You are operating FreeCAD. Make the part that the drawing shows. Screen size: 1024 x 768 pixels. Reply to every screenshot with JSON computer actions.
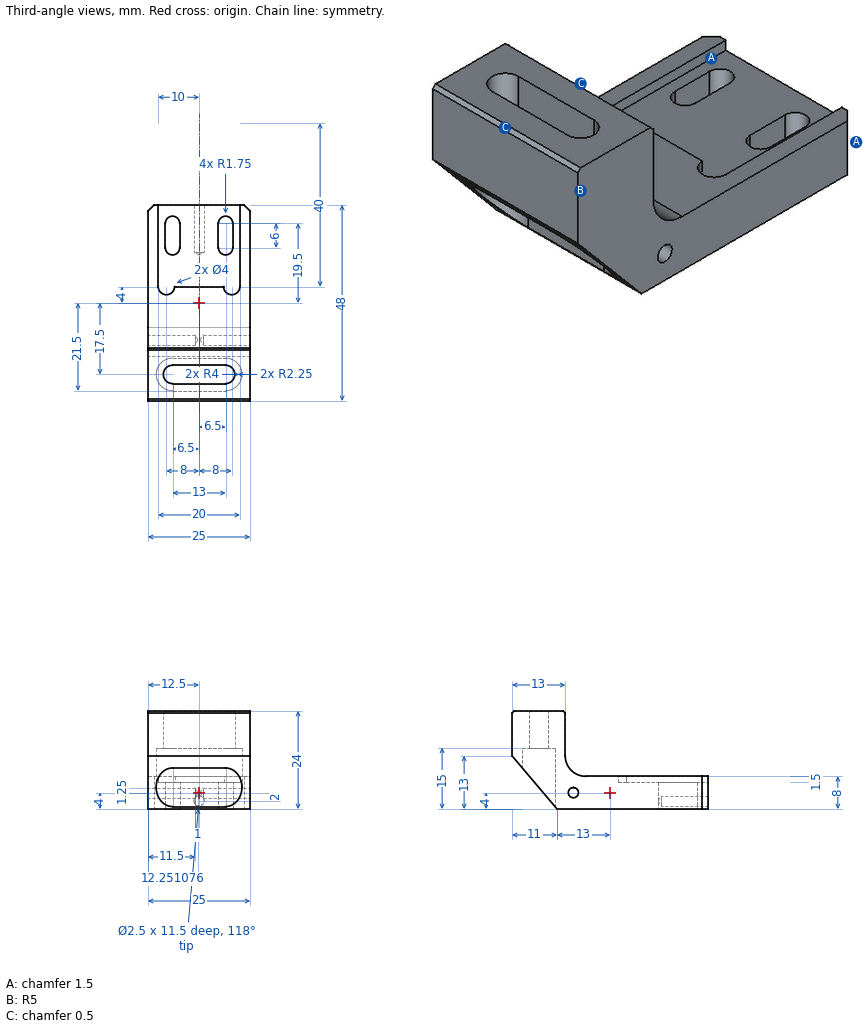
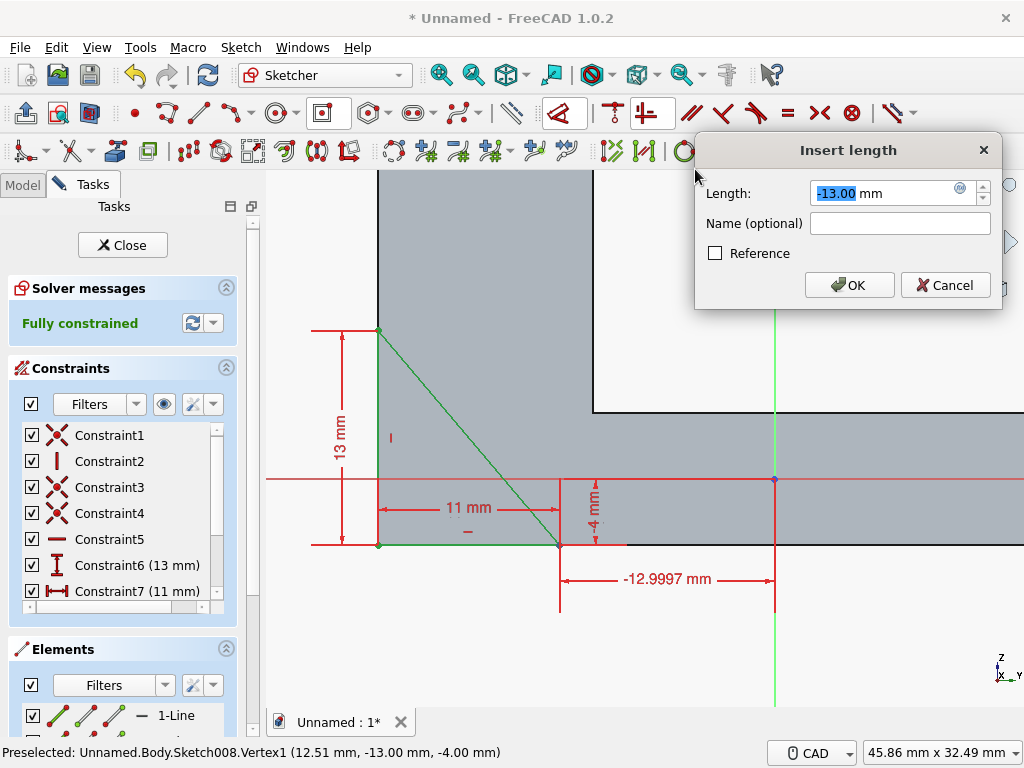
{"action": "type", "text": "-13"}
{"action": "key", "text": "Return"}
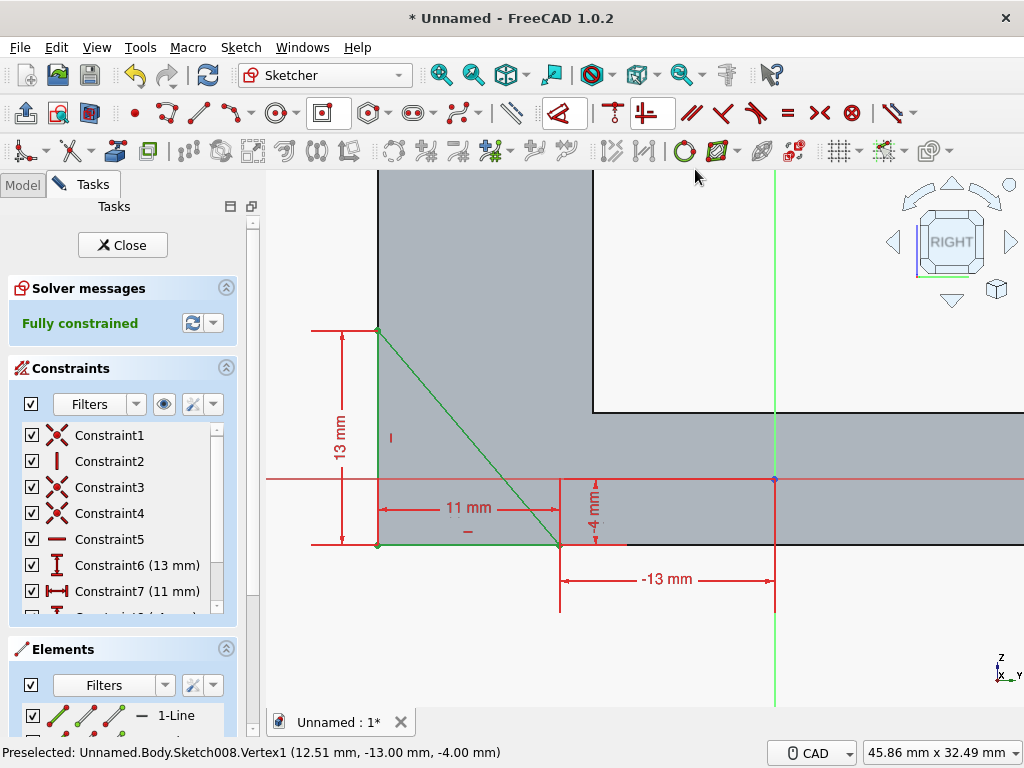
{"action": "left_click", "coordinate": [123, 245]}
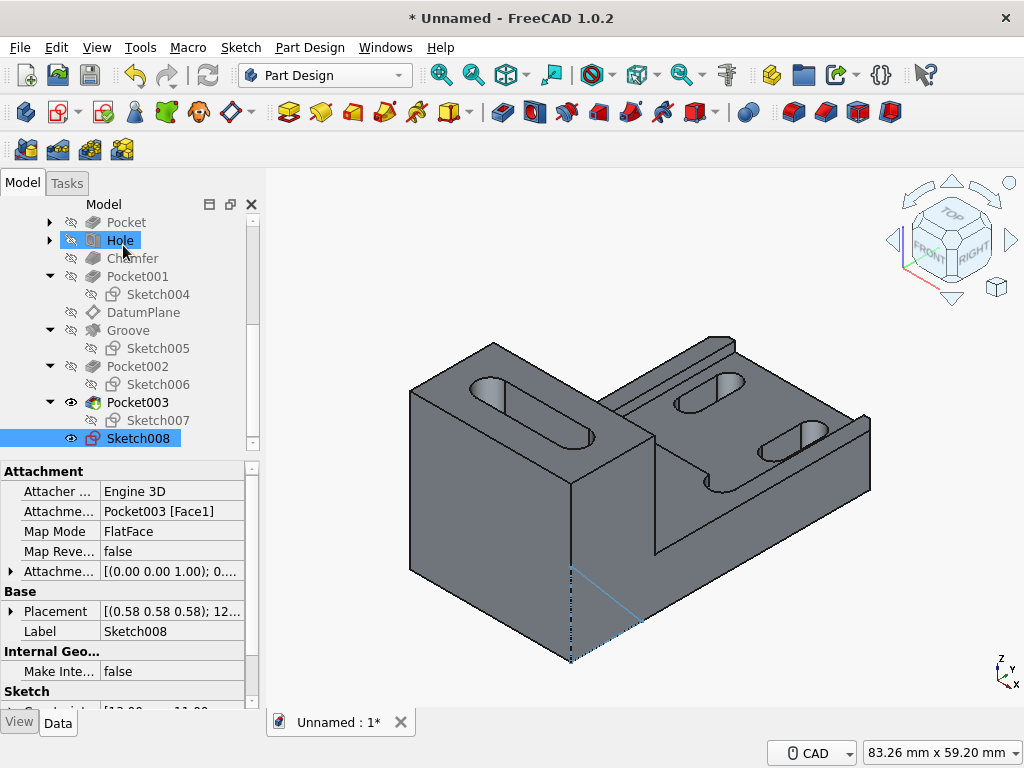
{"action": "left_click", "coordinate": [504, 112]}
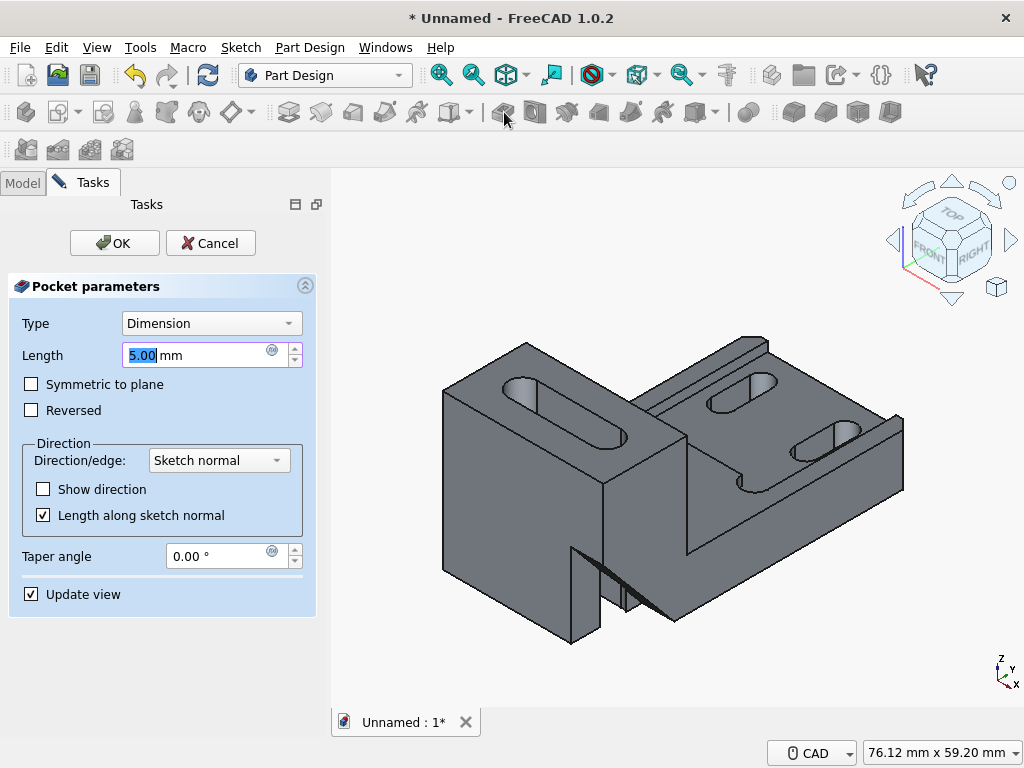
{"action": "left_click", "coordinate": [212, 324]}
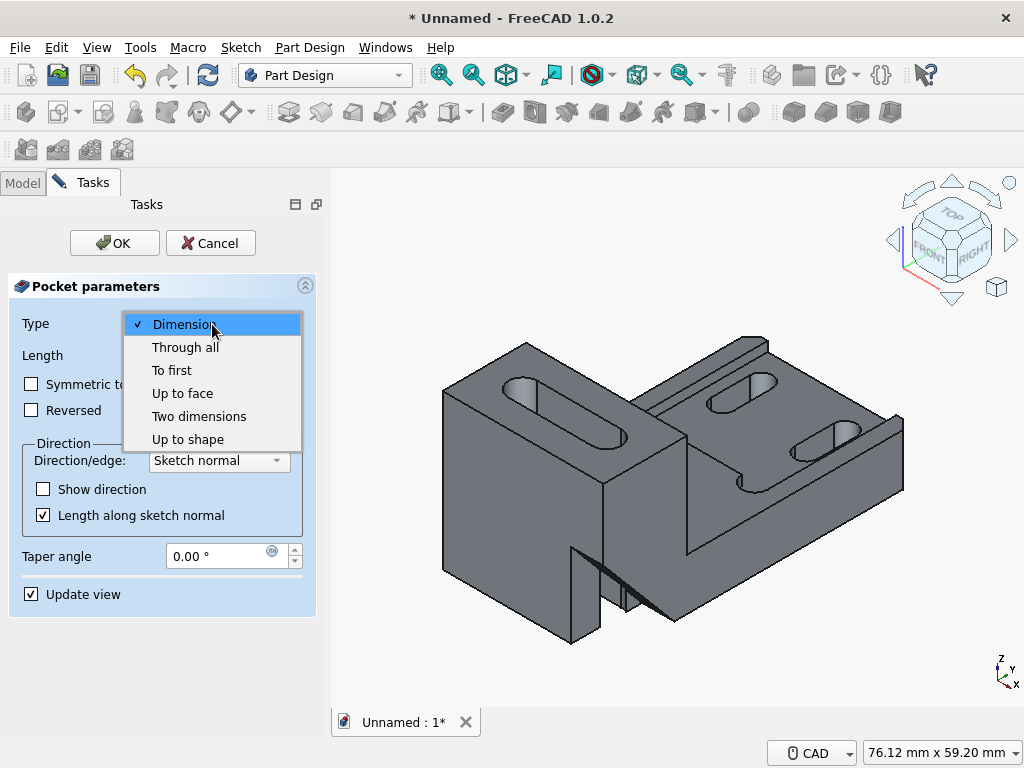
{"action": "left_click", "coordinate": [212, 348]}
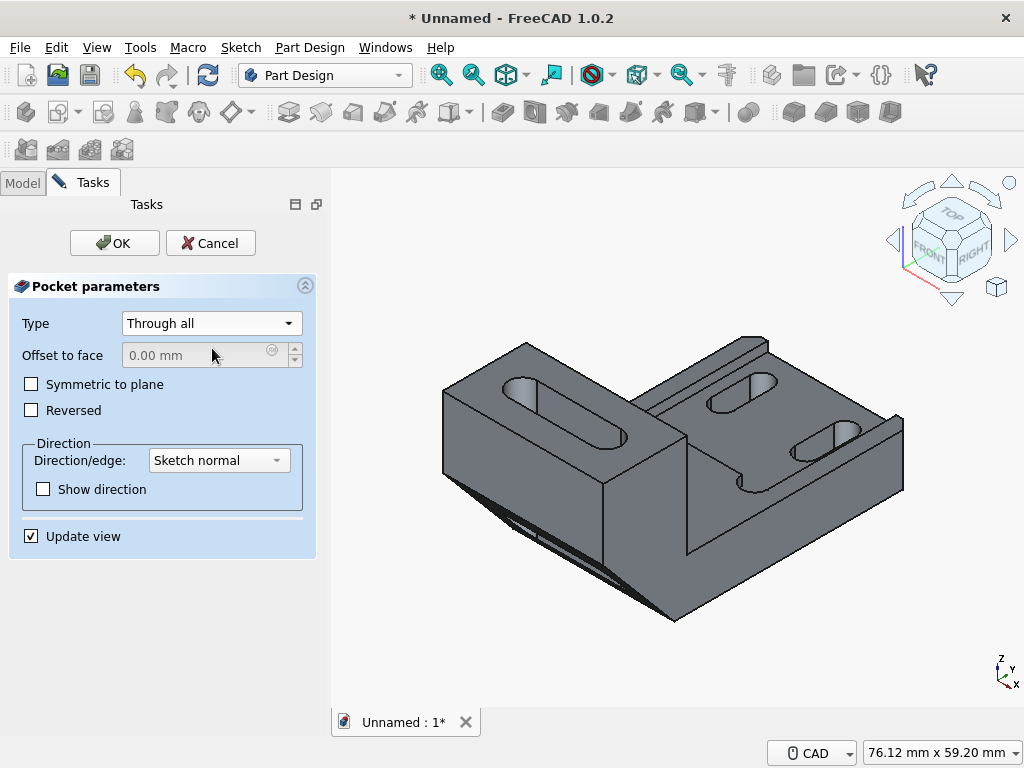
{"action": "left_click", "coordinate": [115, 243]}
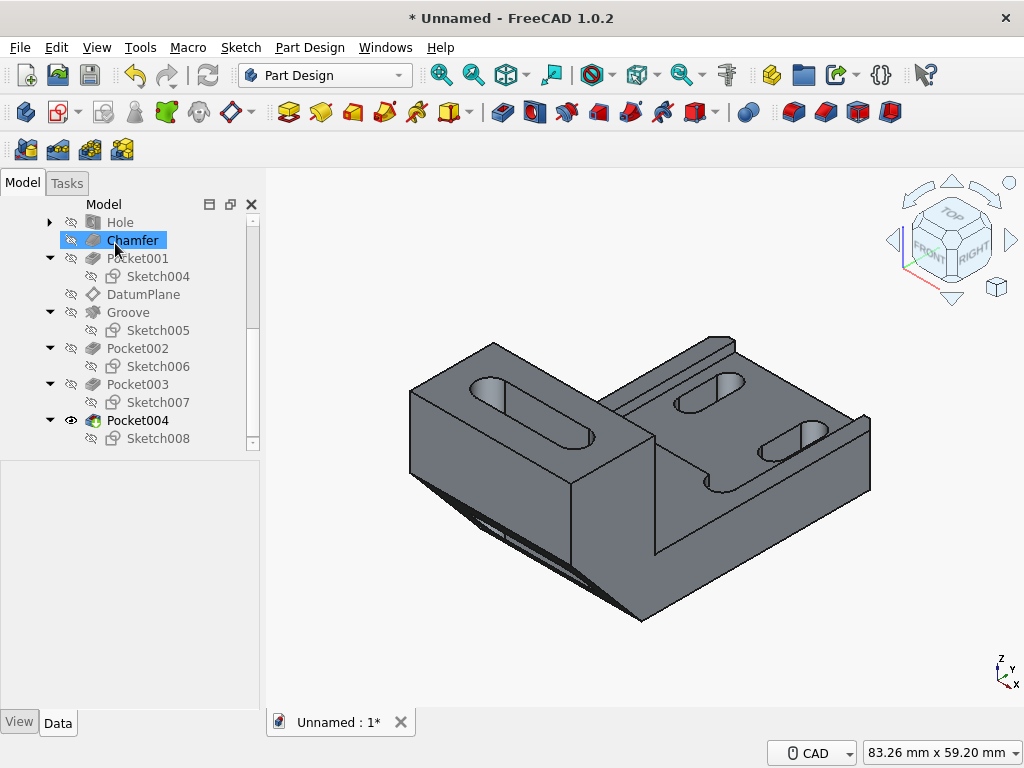
{"action": "key", "text": "5"}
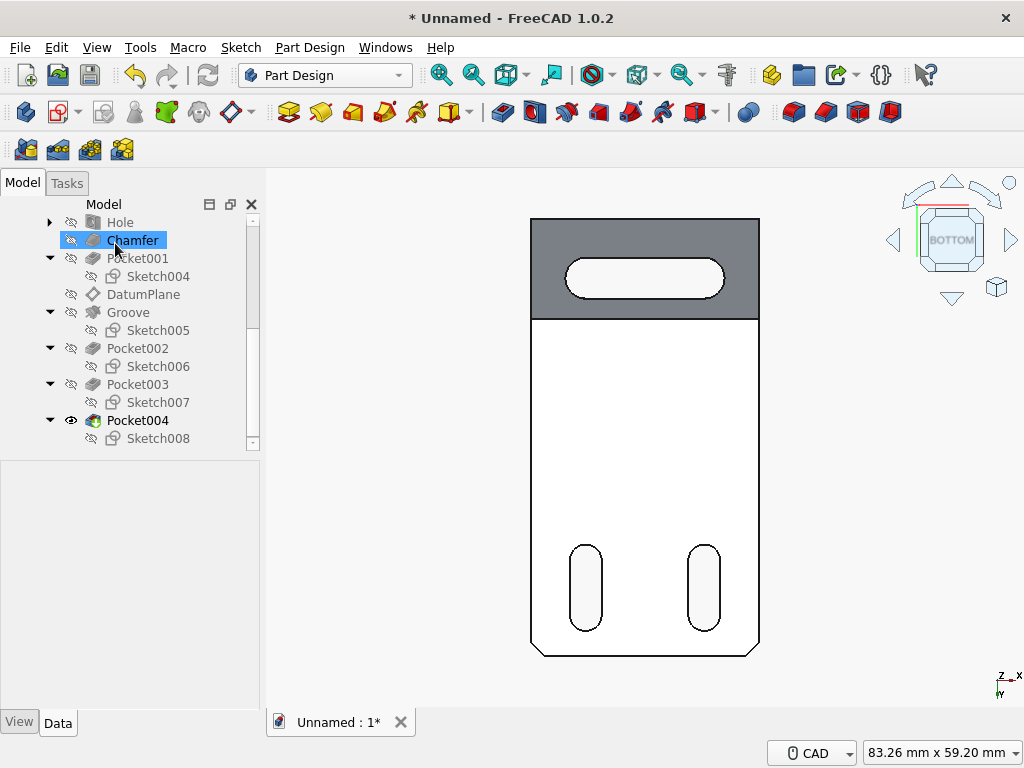
{"action": "left_click", "coordinate": [645, 438]}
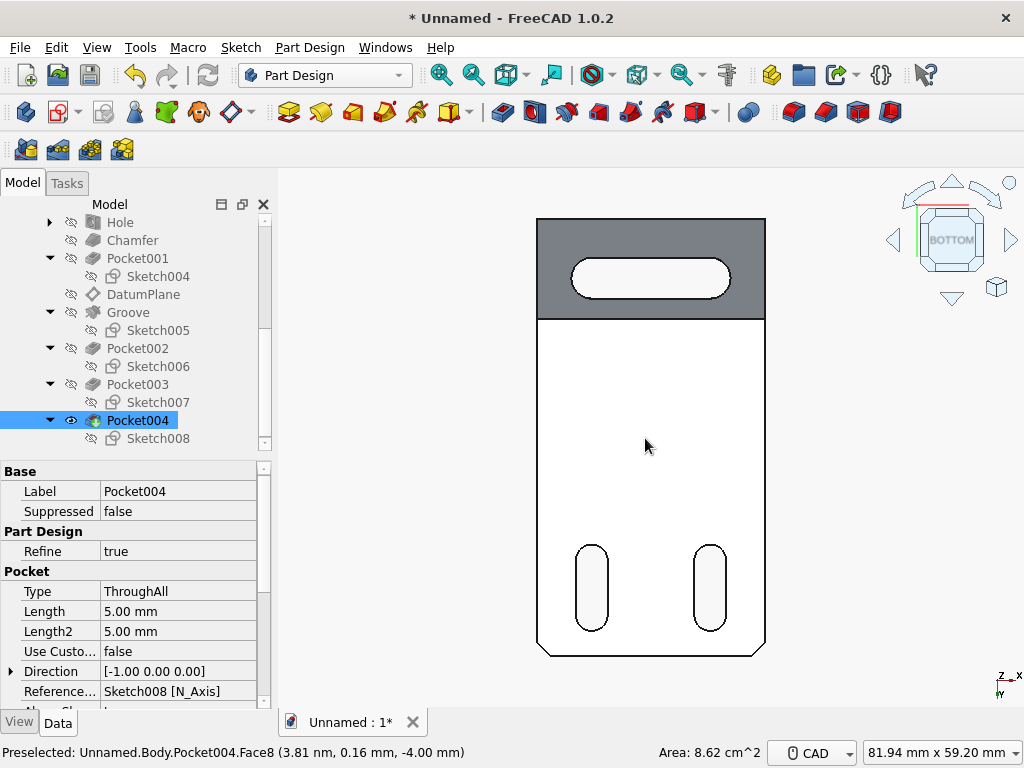
{"action": "left_click", "coordinate": [58, 112]}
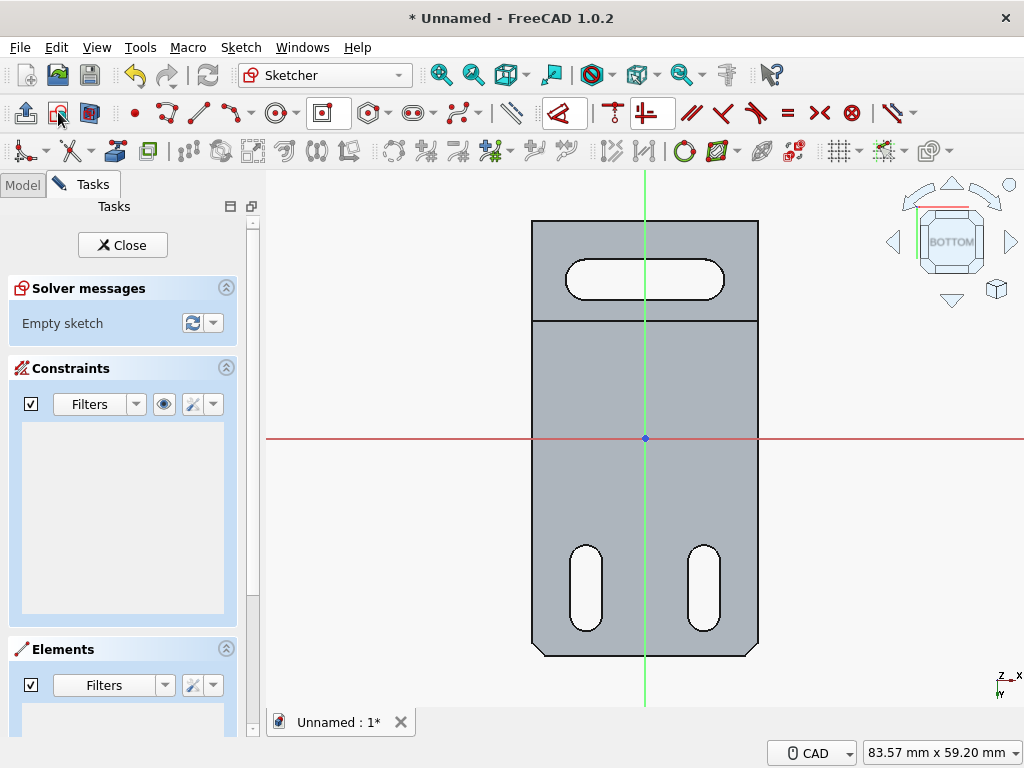
{"action": "scroll", "coordinate": [728, 222], "scroll_direction": "up", "scroll_amount": 3}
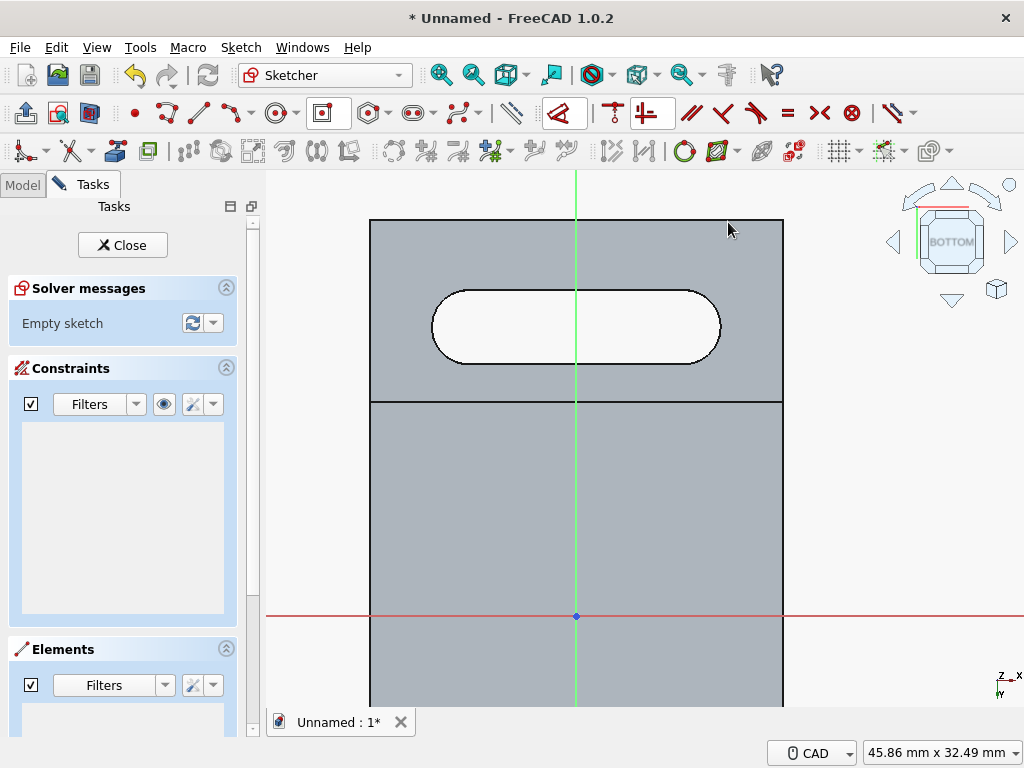
{"action": "left_click", "coordinate": [414, 114]}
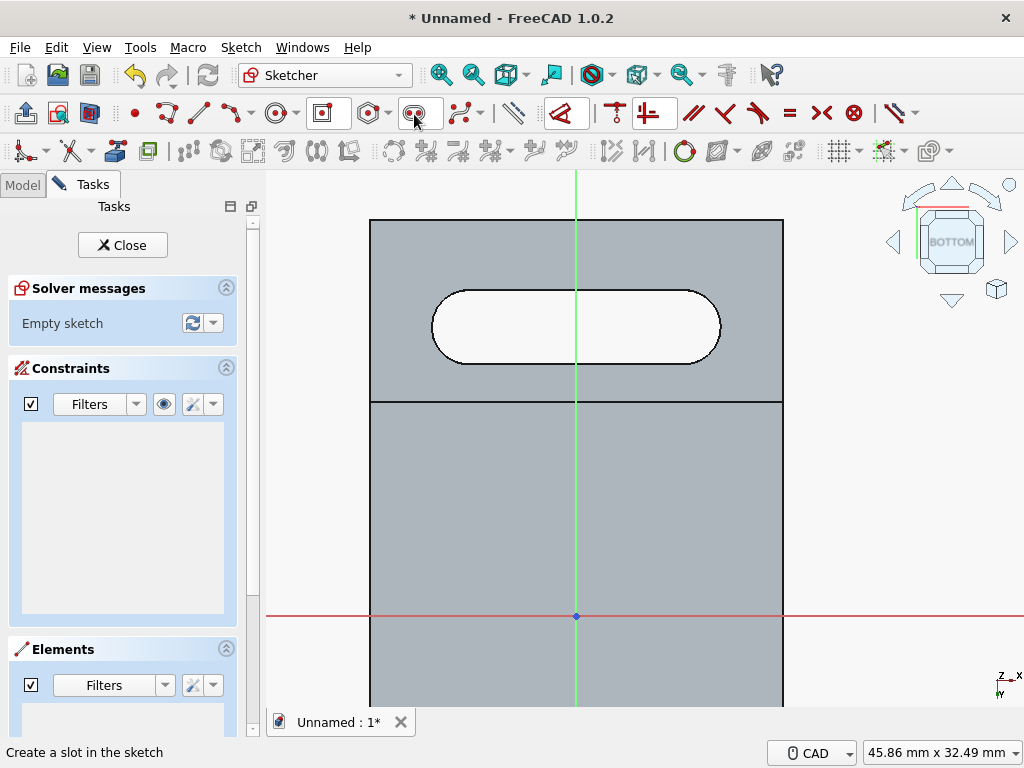
{"action": "left_click", "coordinate": [469, 327]}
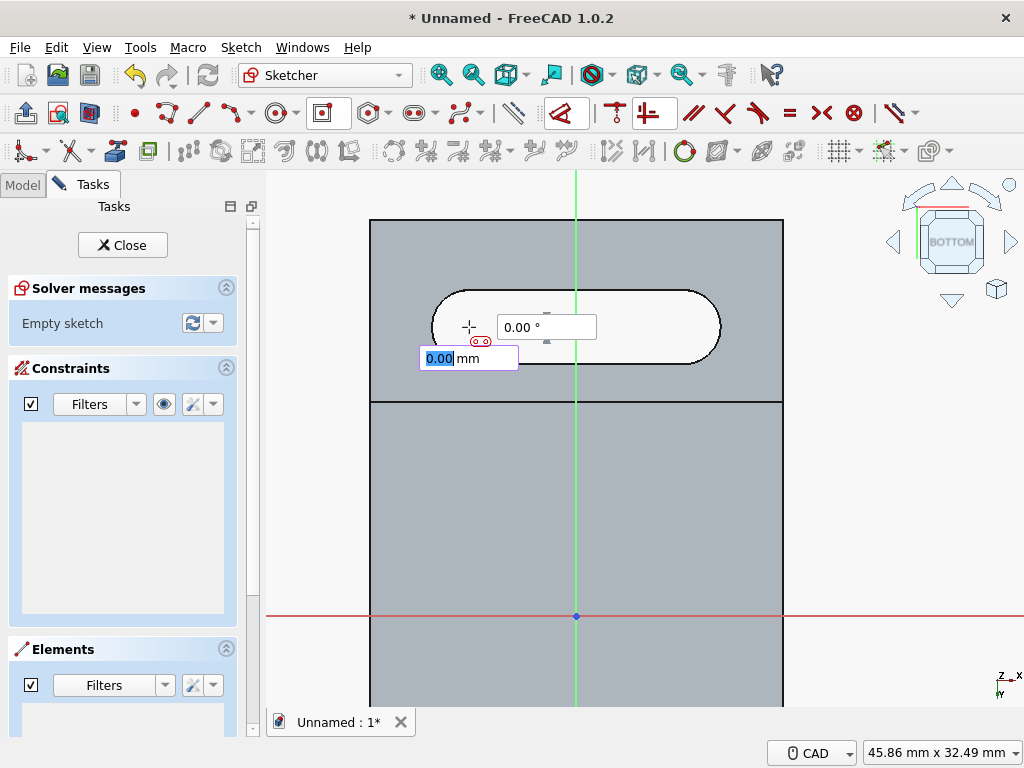
{"action": "left_click", "coordinate": [684, 327]}